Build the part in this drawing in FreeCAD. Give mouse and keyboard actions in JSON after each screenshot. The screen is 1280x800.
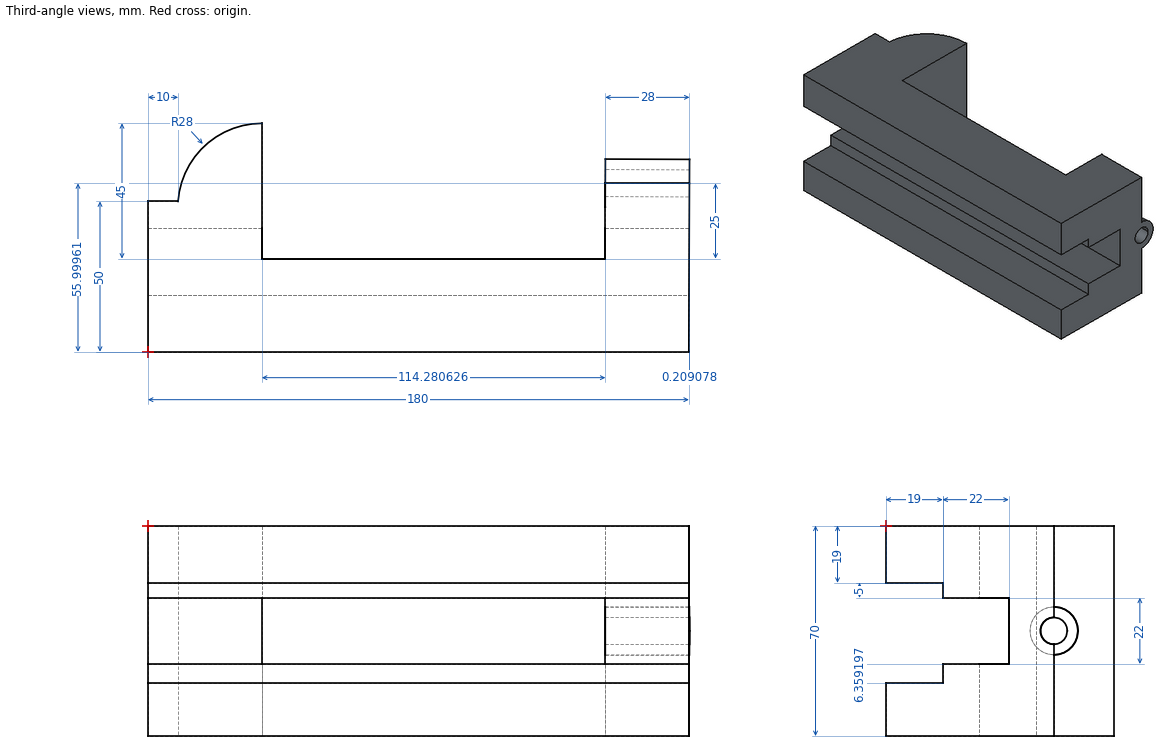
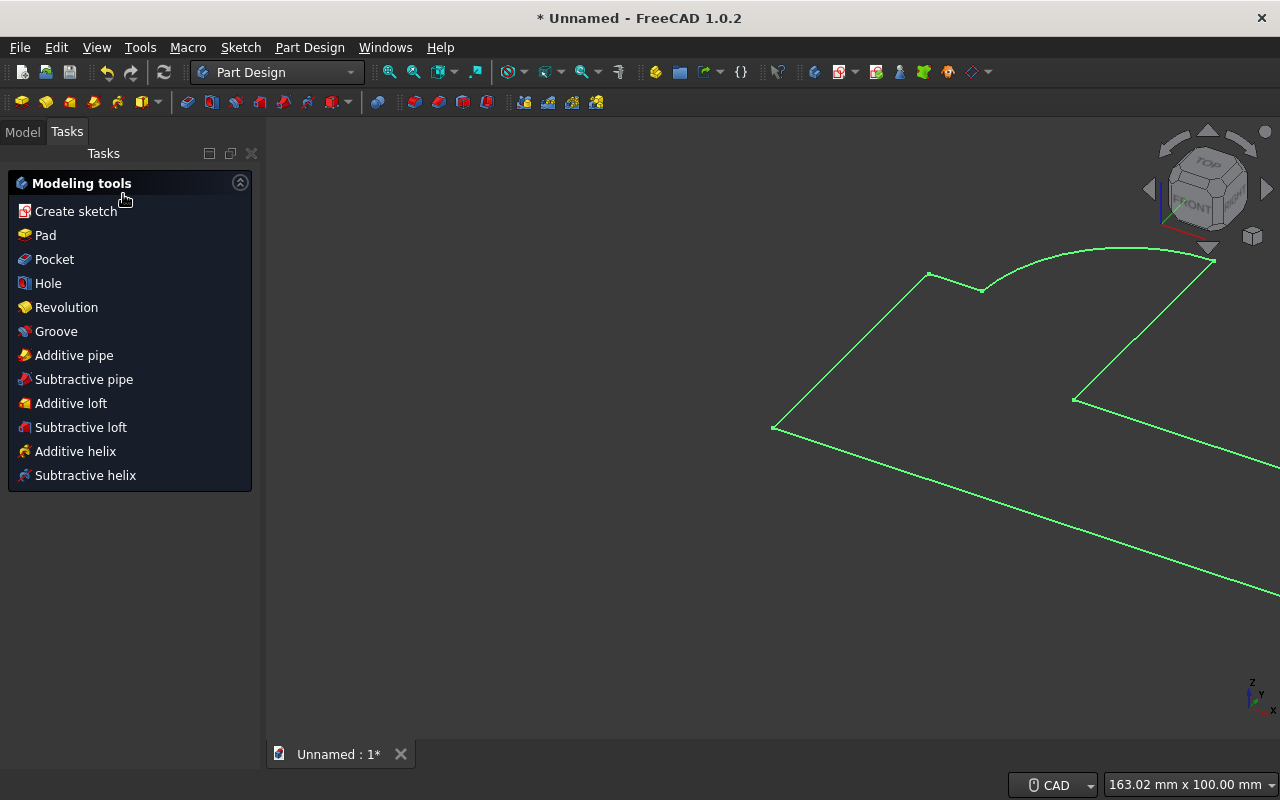
{"action": "left_click", "coordinate": [22, 102]}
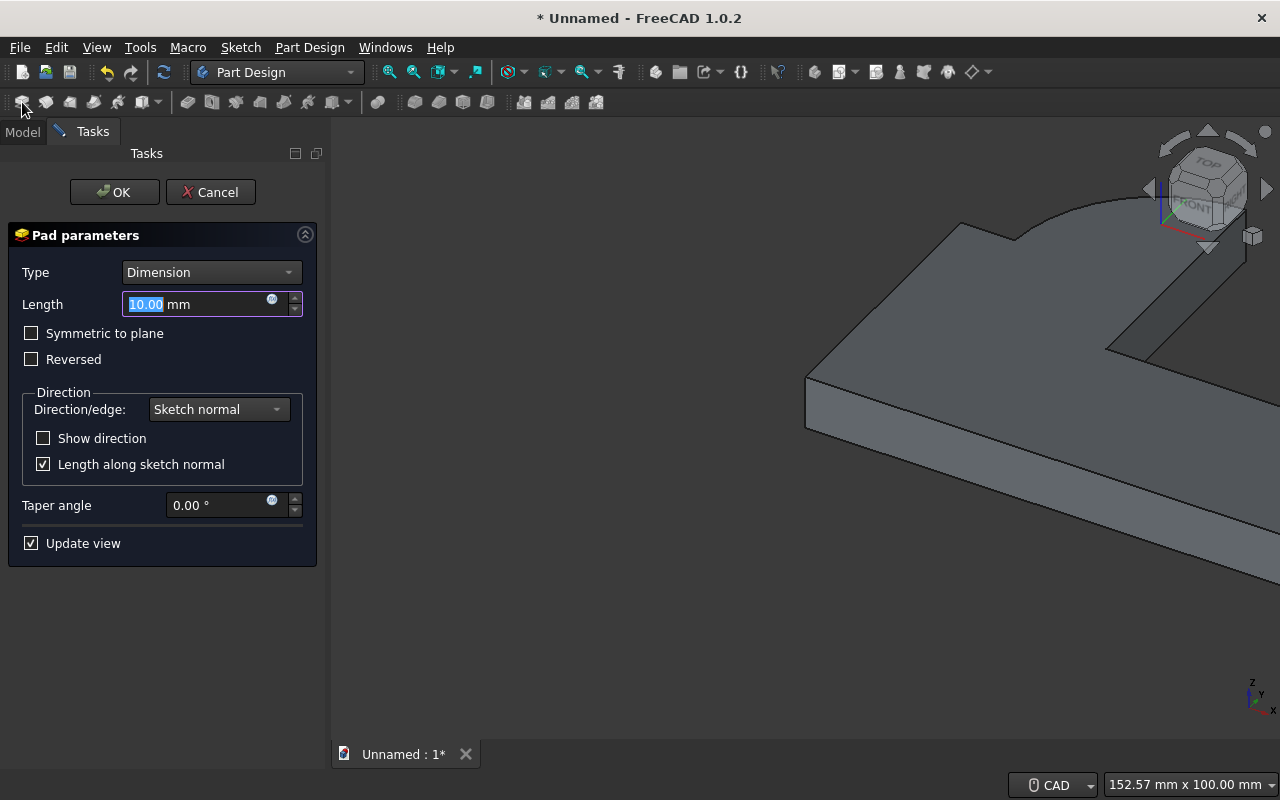
{"action": "type", "text": "70"}
{"action": "key", "text": "Tab"}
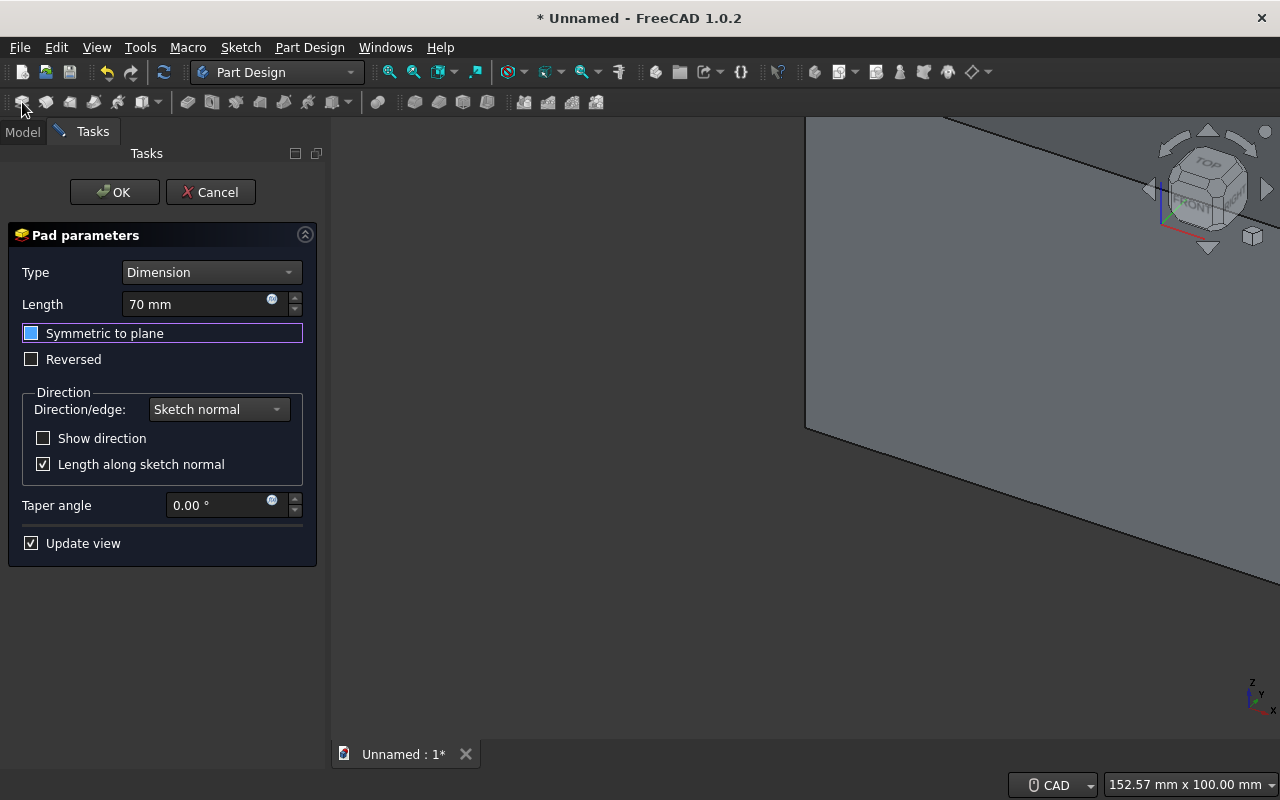
{"action": "left_click", "coordinate": [30, 359]}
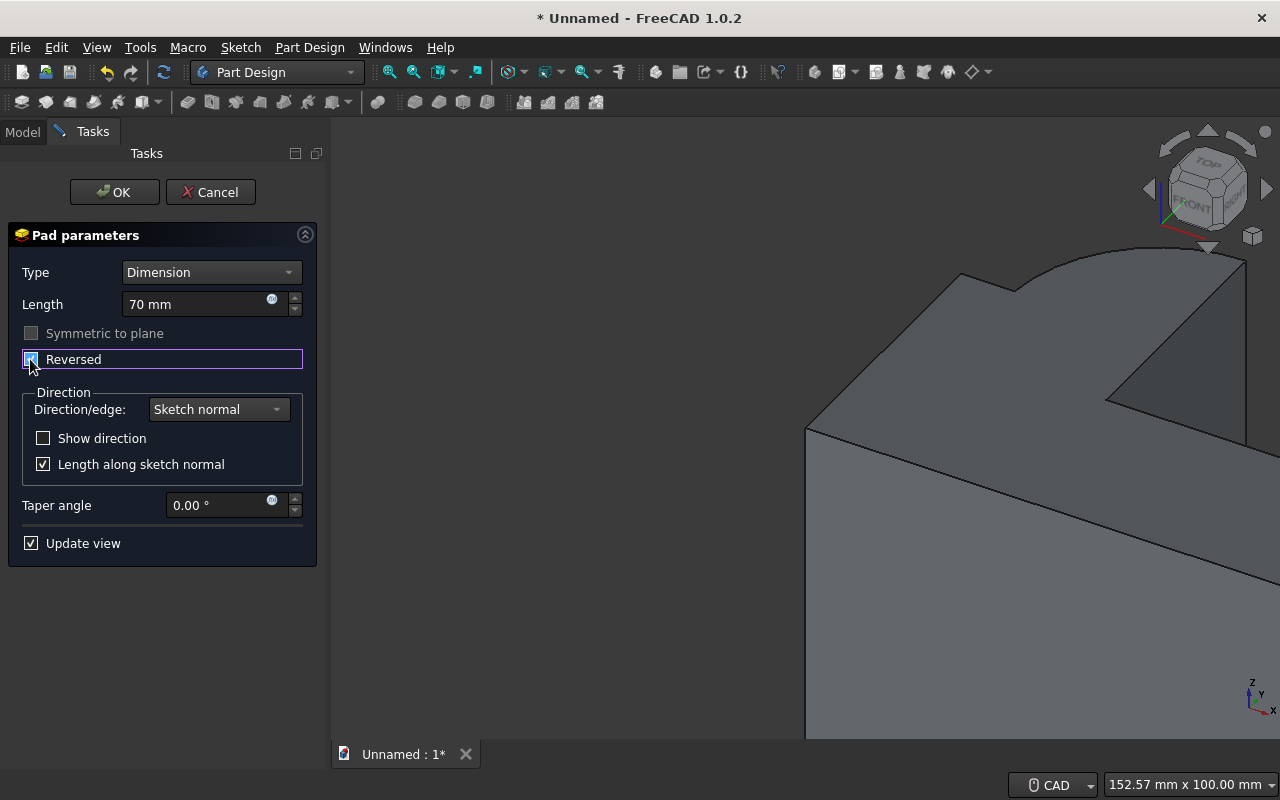
{"action": "left_click", "coordinate": [115, 192]}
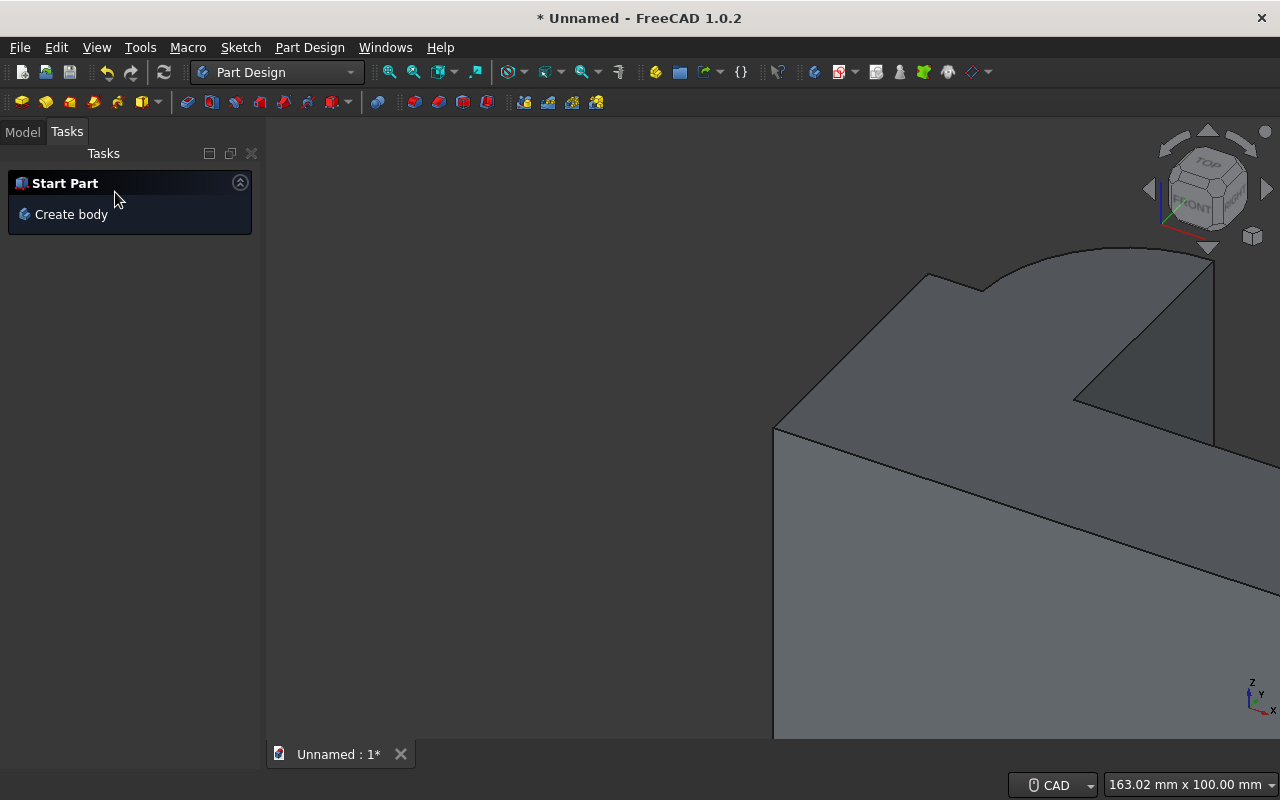
{"action": "left_click", "coordinate": [390, 72]}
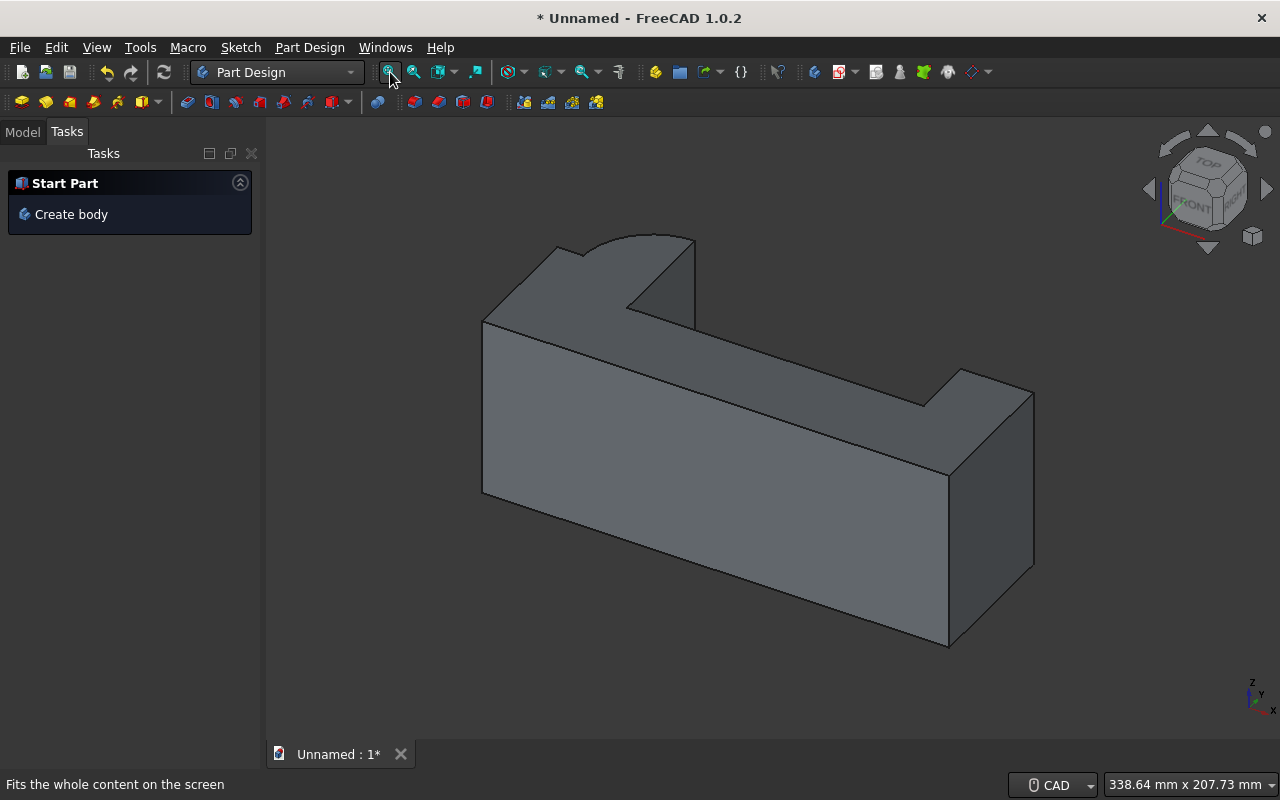
{"action": "left_click", "coordinate": [991, 519]}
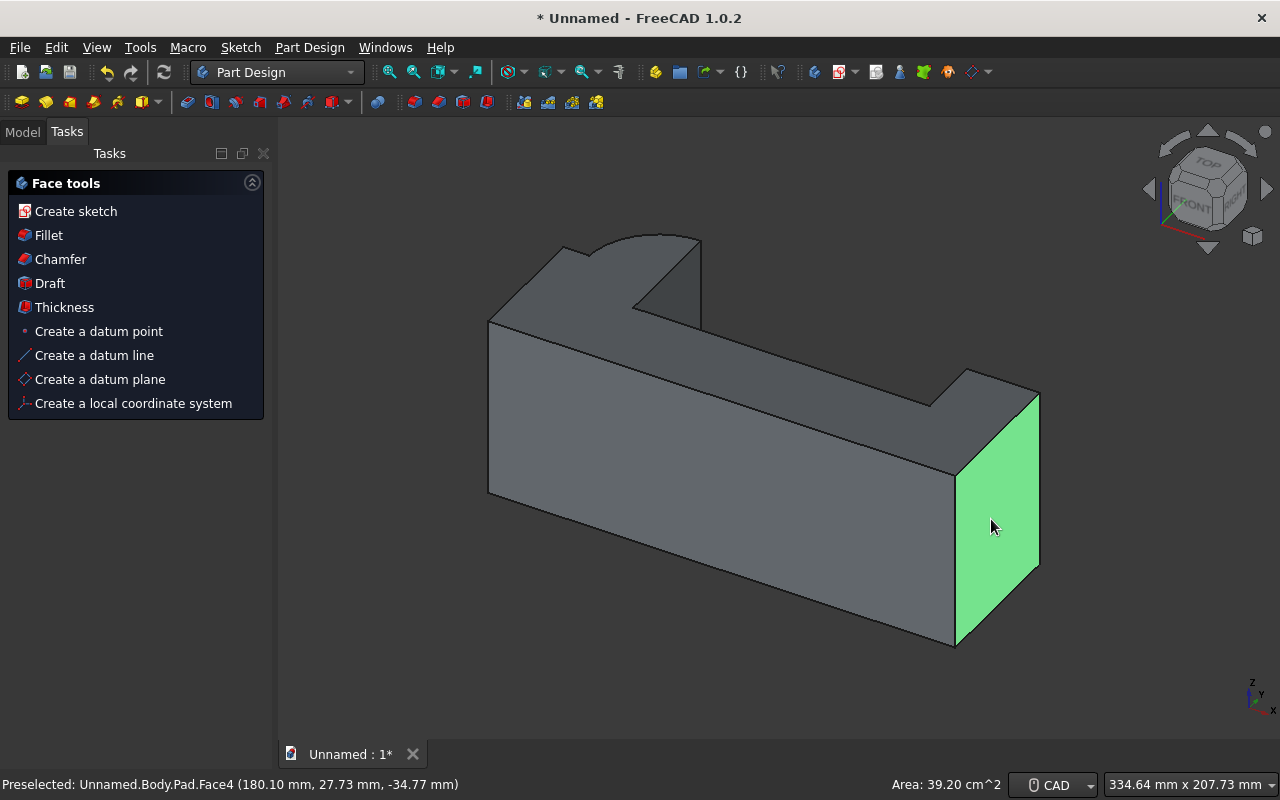
{"action": "left_click", "coordinate": [840, 72]}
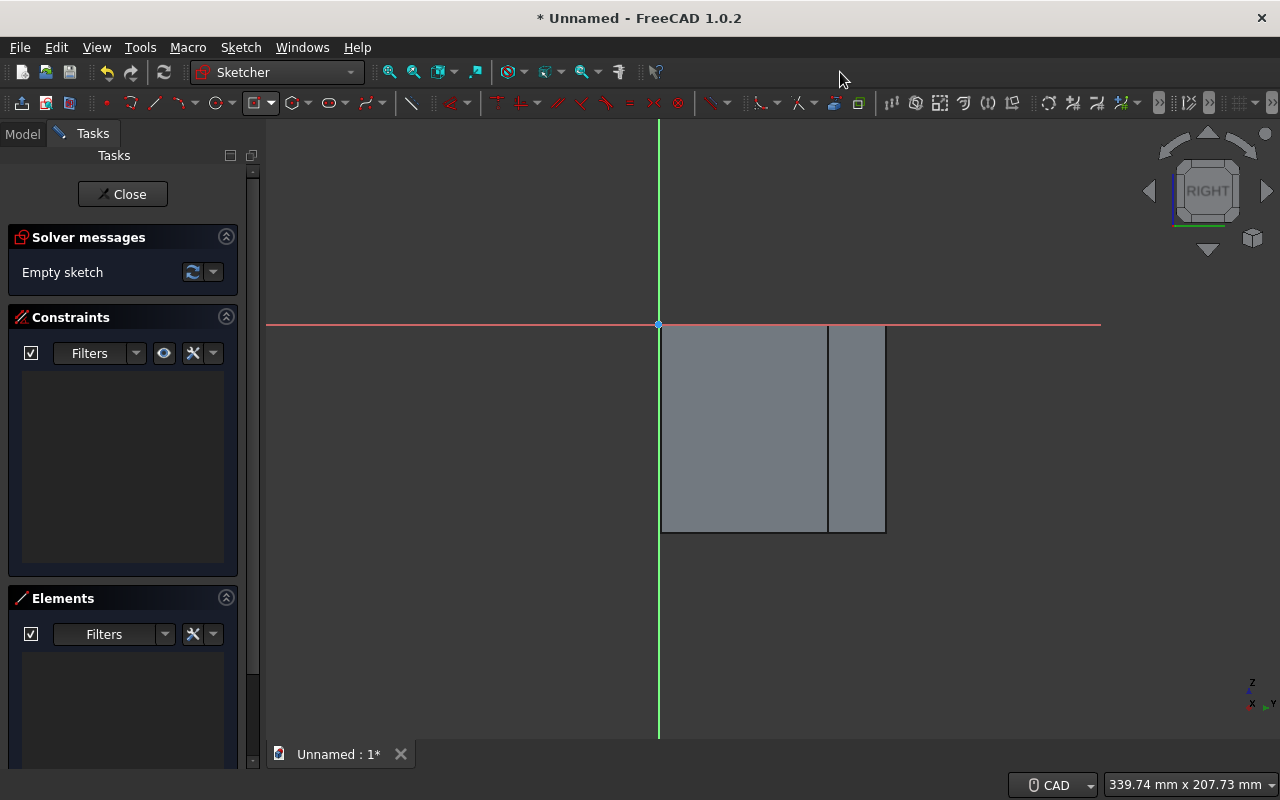
{"action": "left_click", "coordinate": [70, 104]}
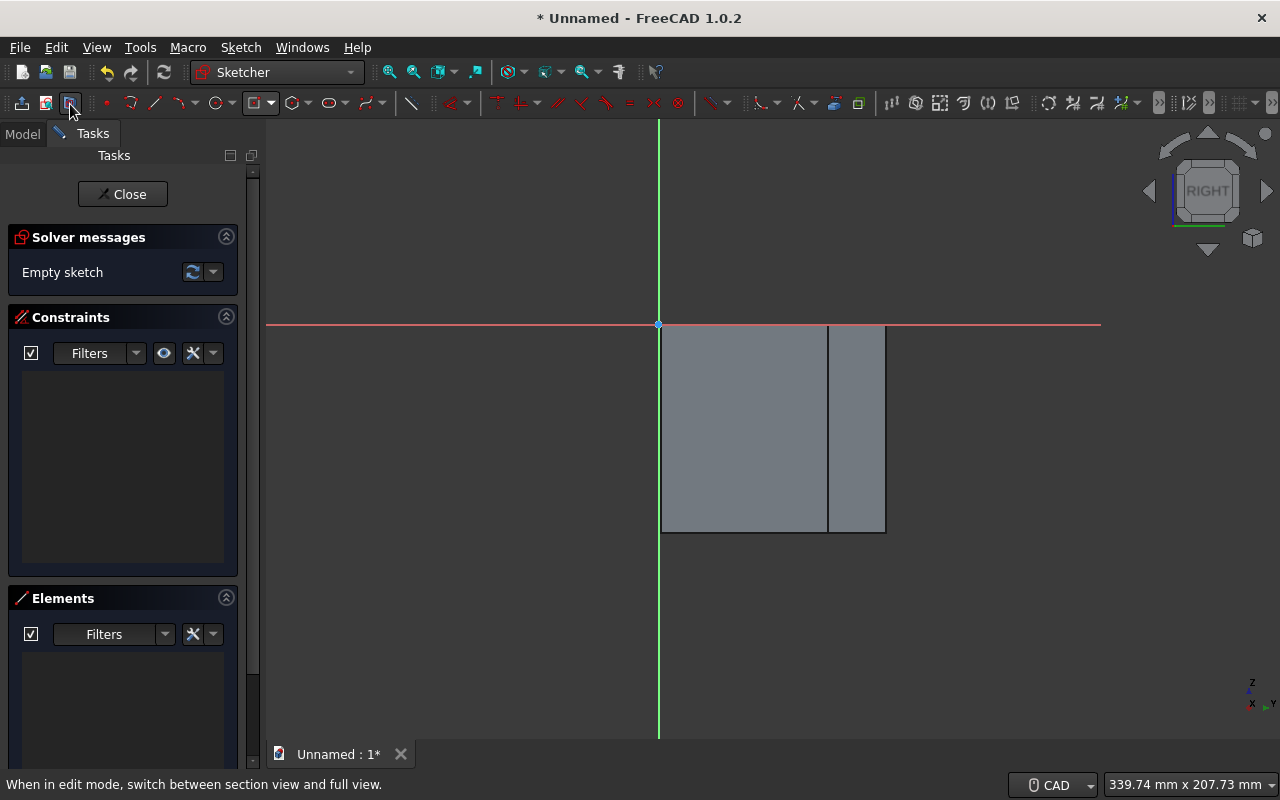
{"action": "scroll", "coordinate": [843, 429], "scroll_direction": "up", "scroll_amount": 11}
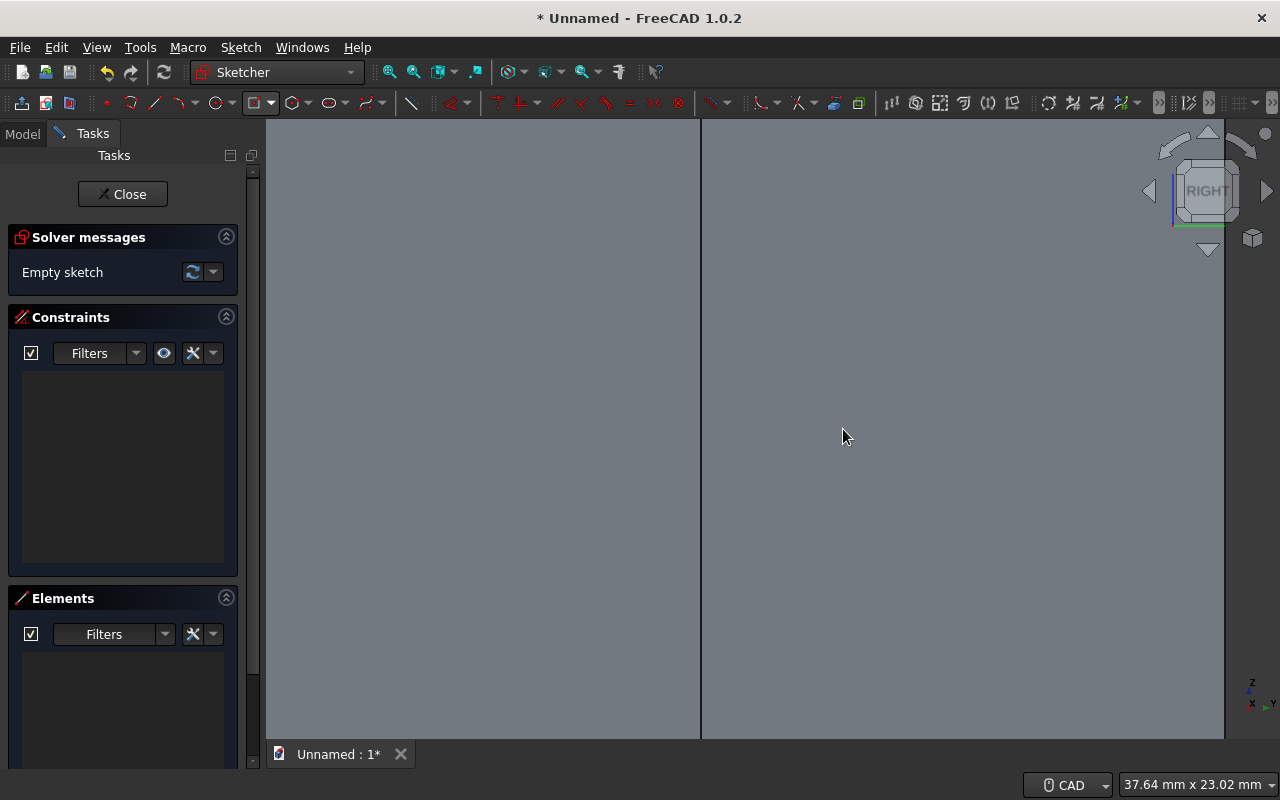
{"action": "left_click", "coordinate": [216, 104]}